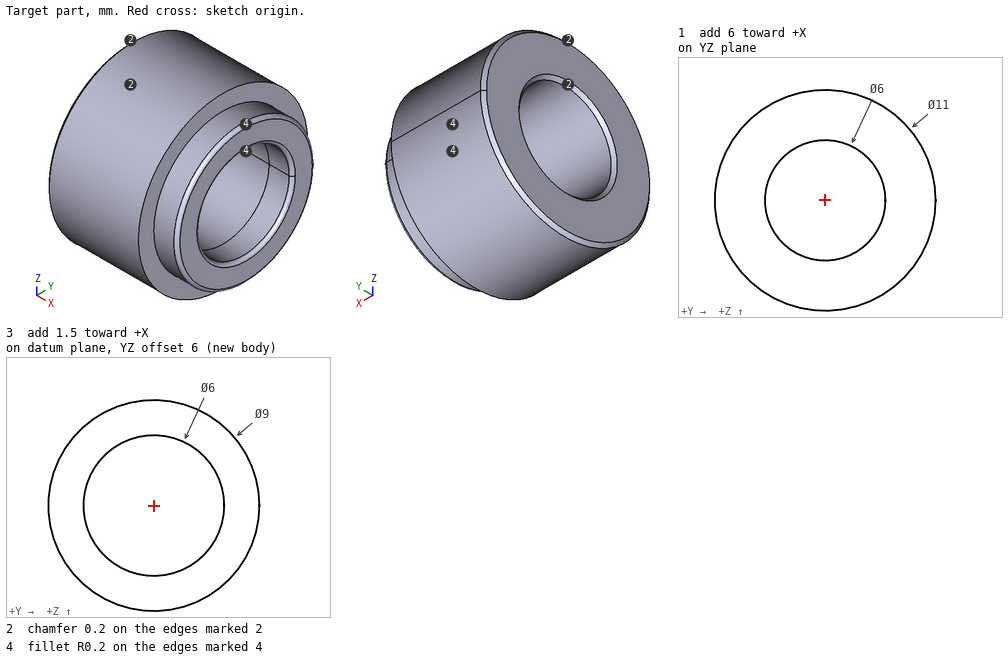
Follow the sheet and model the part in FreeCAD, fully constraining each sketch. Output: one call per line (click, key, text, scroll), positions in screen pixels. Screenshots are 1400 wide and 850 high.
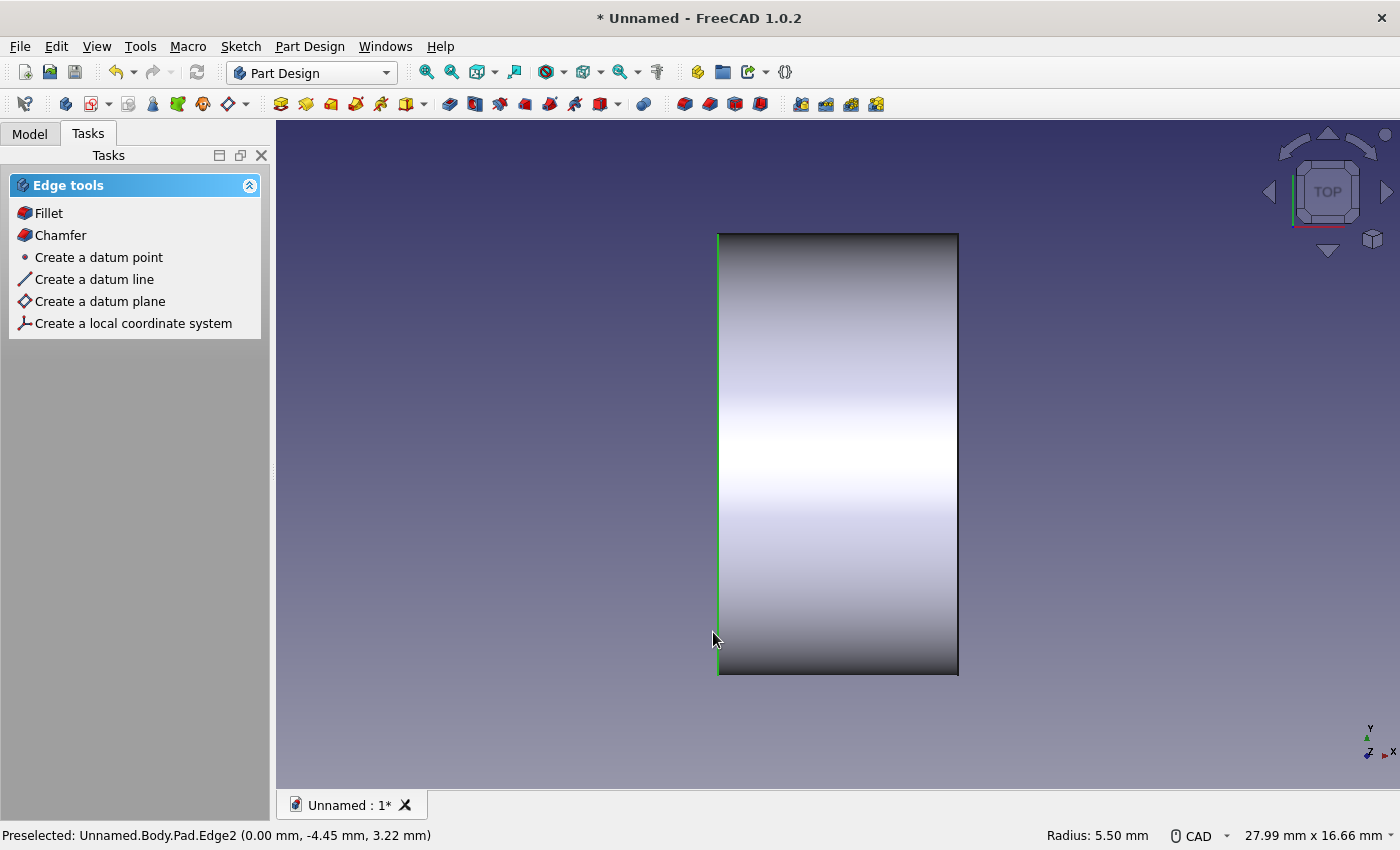
key(1)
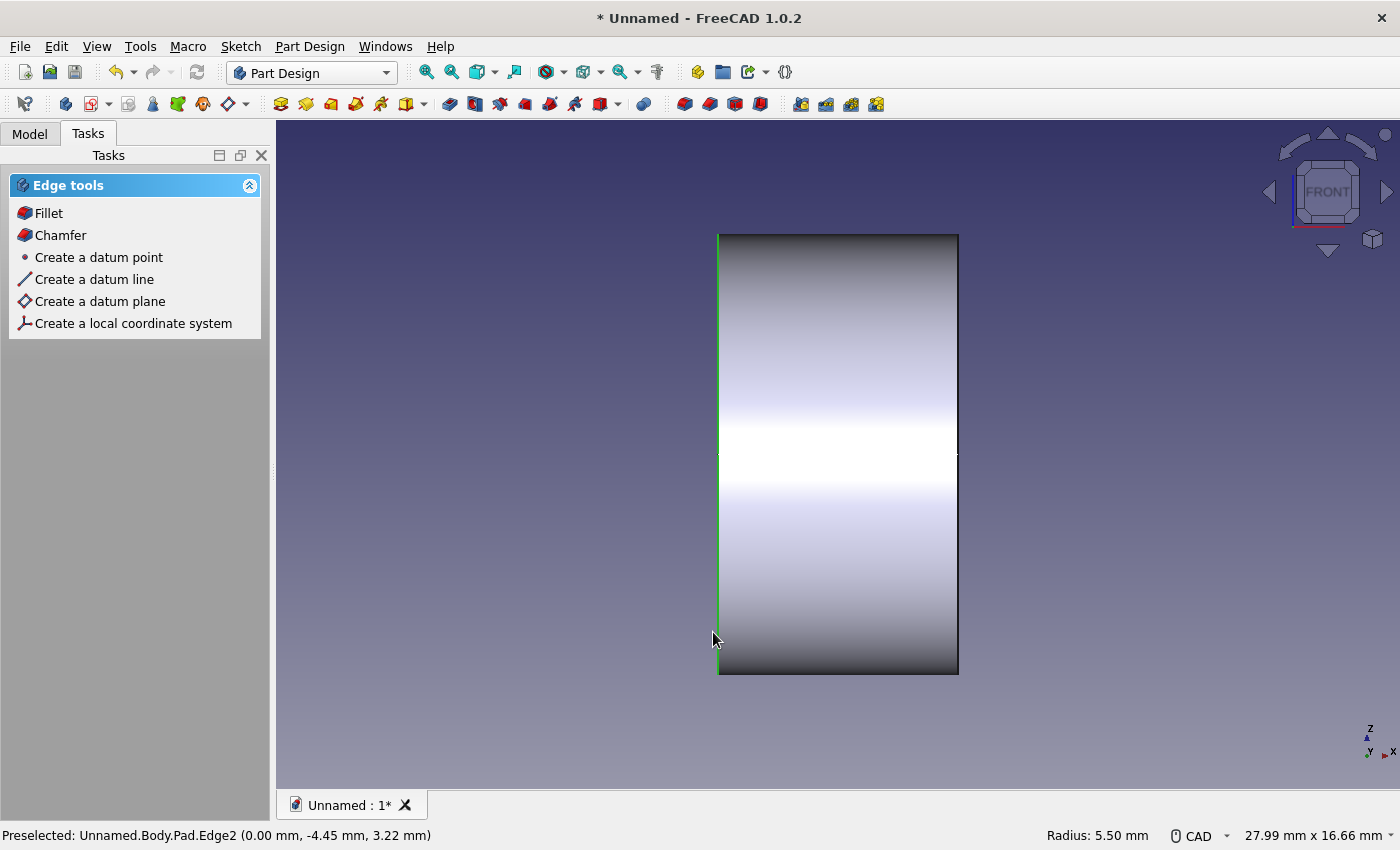
key(3)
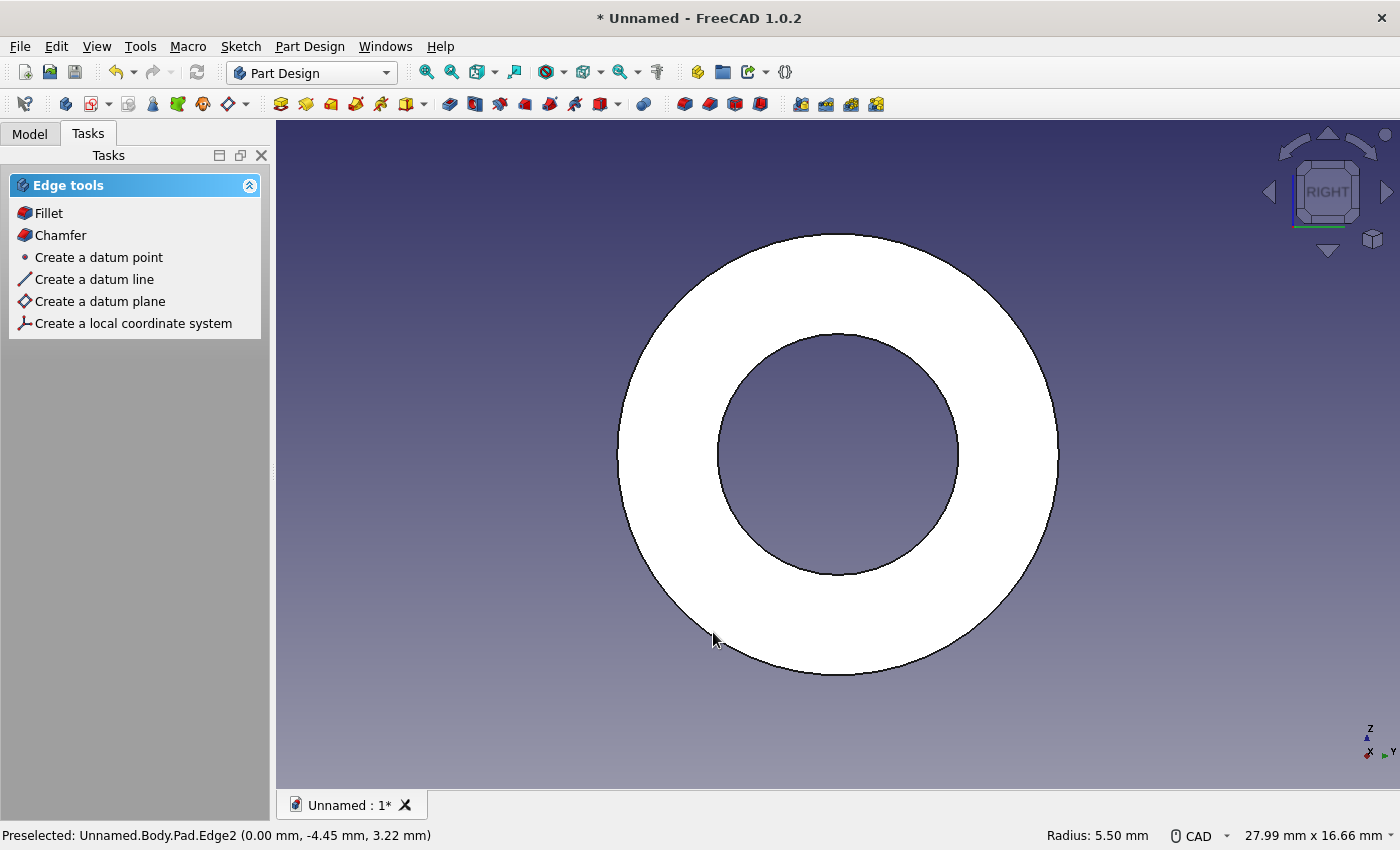
key(5)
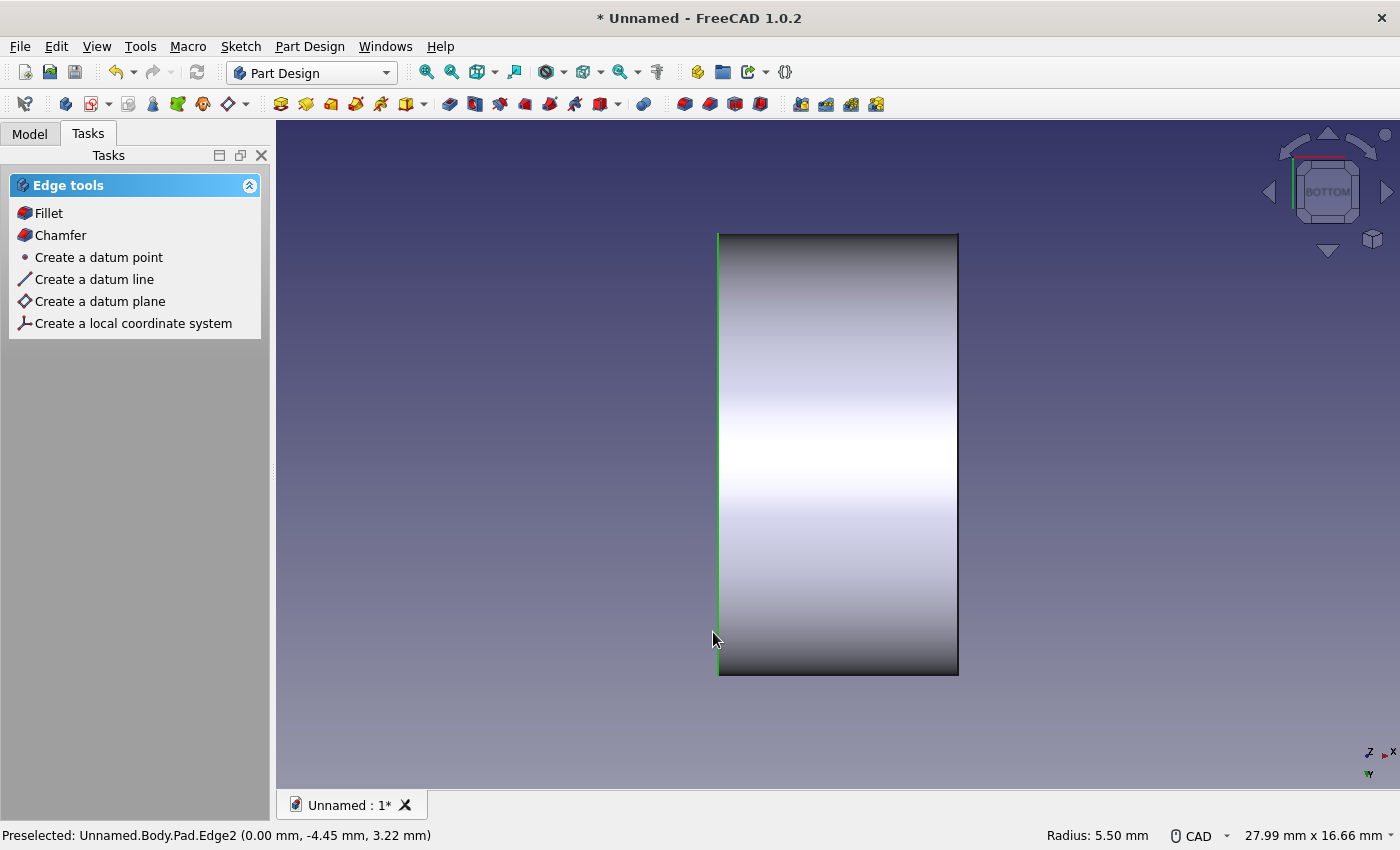
key(4)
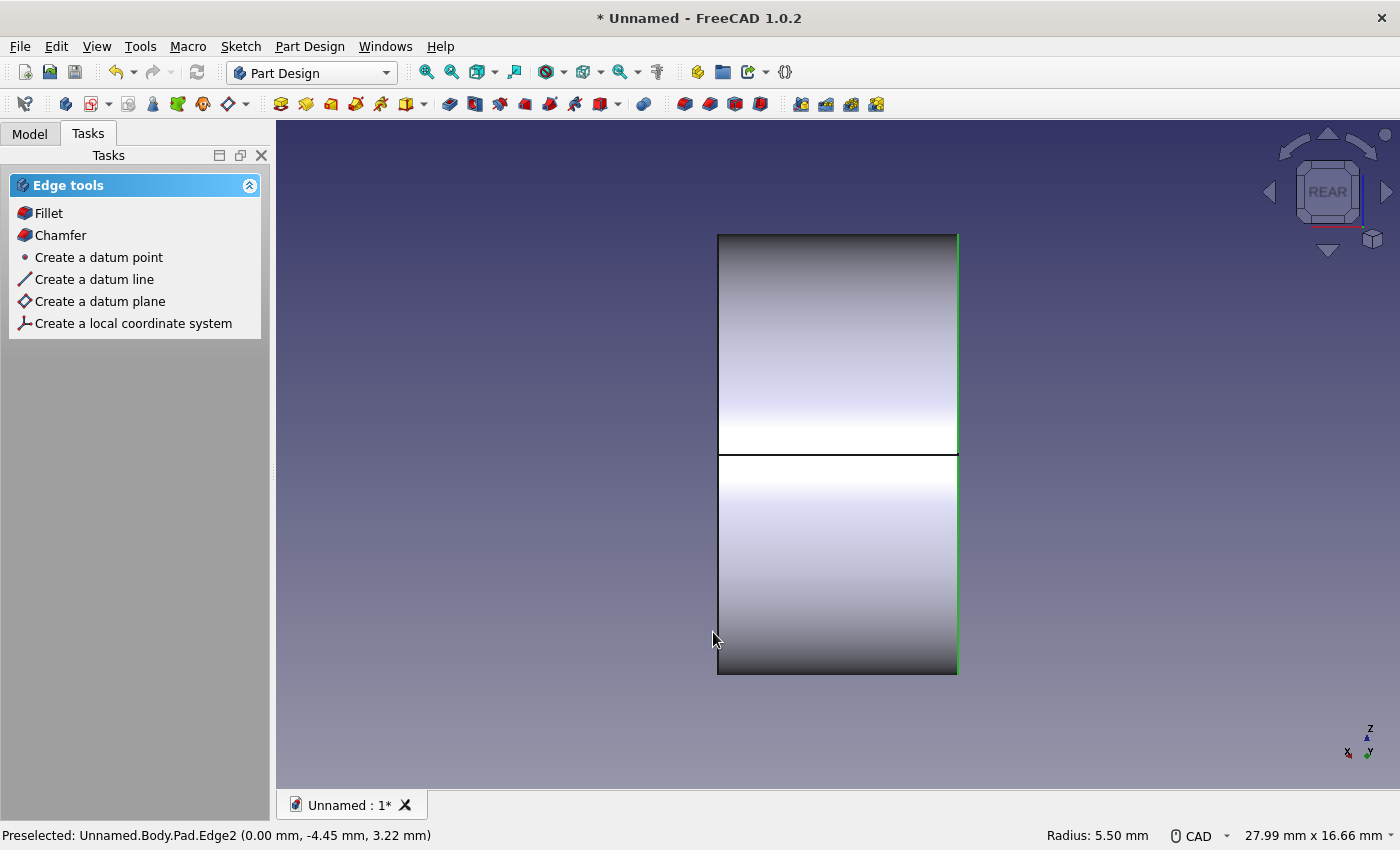
key(6)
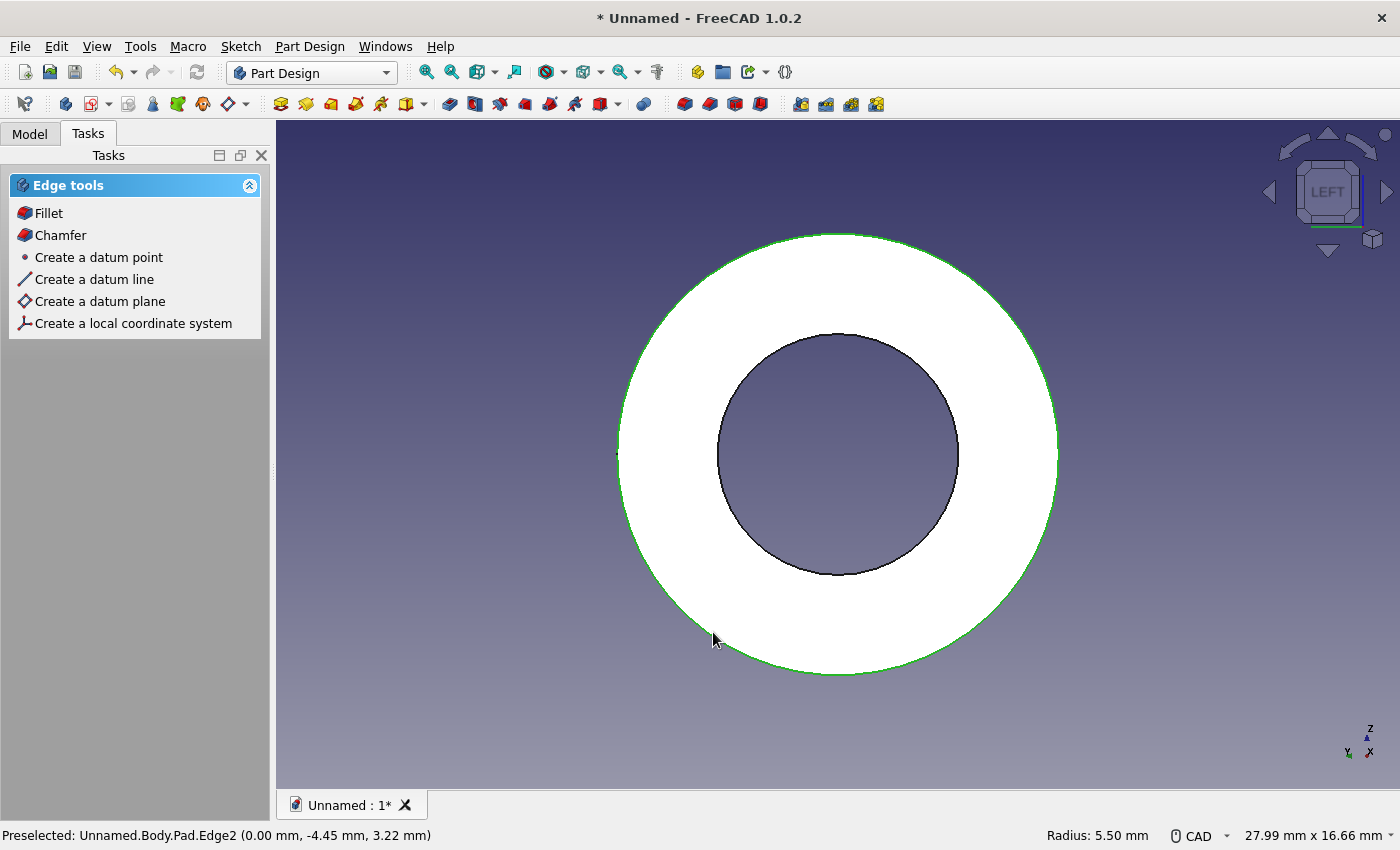
click(958, 453, ctrl)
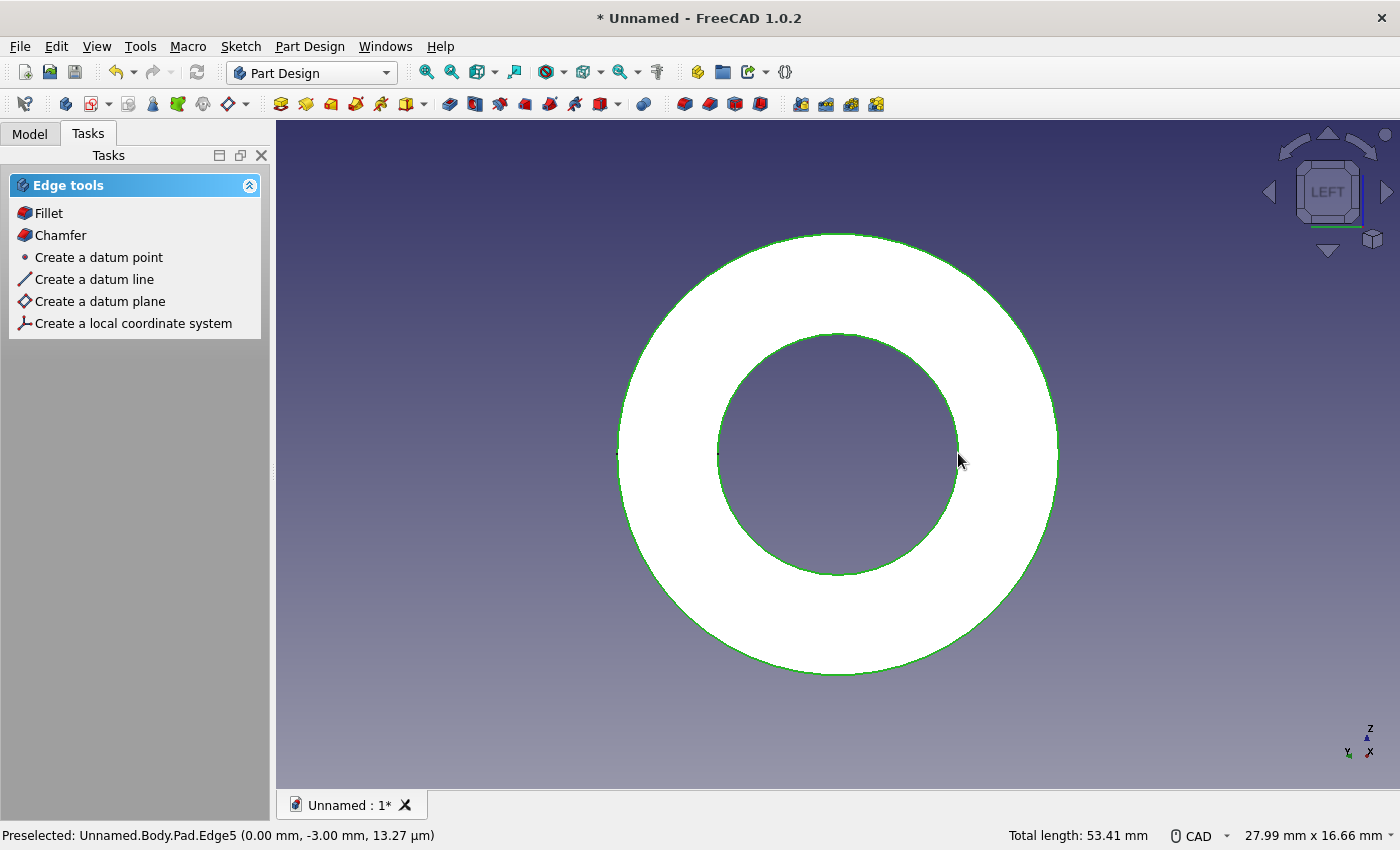
click(710, 104)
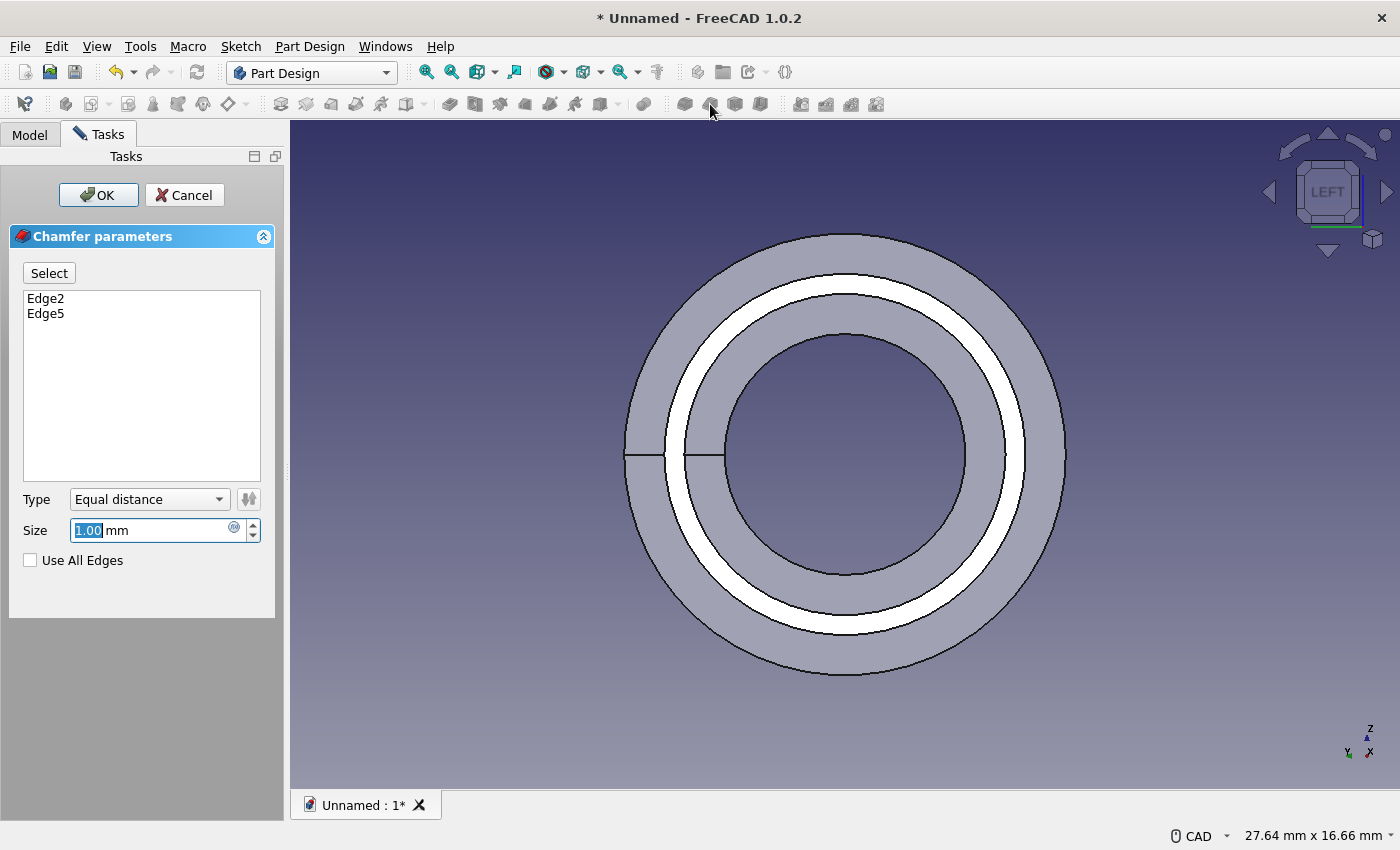
text(0.2)
key(Tab)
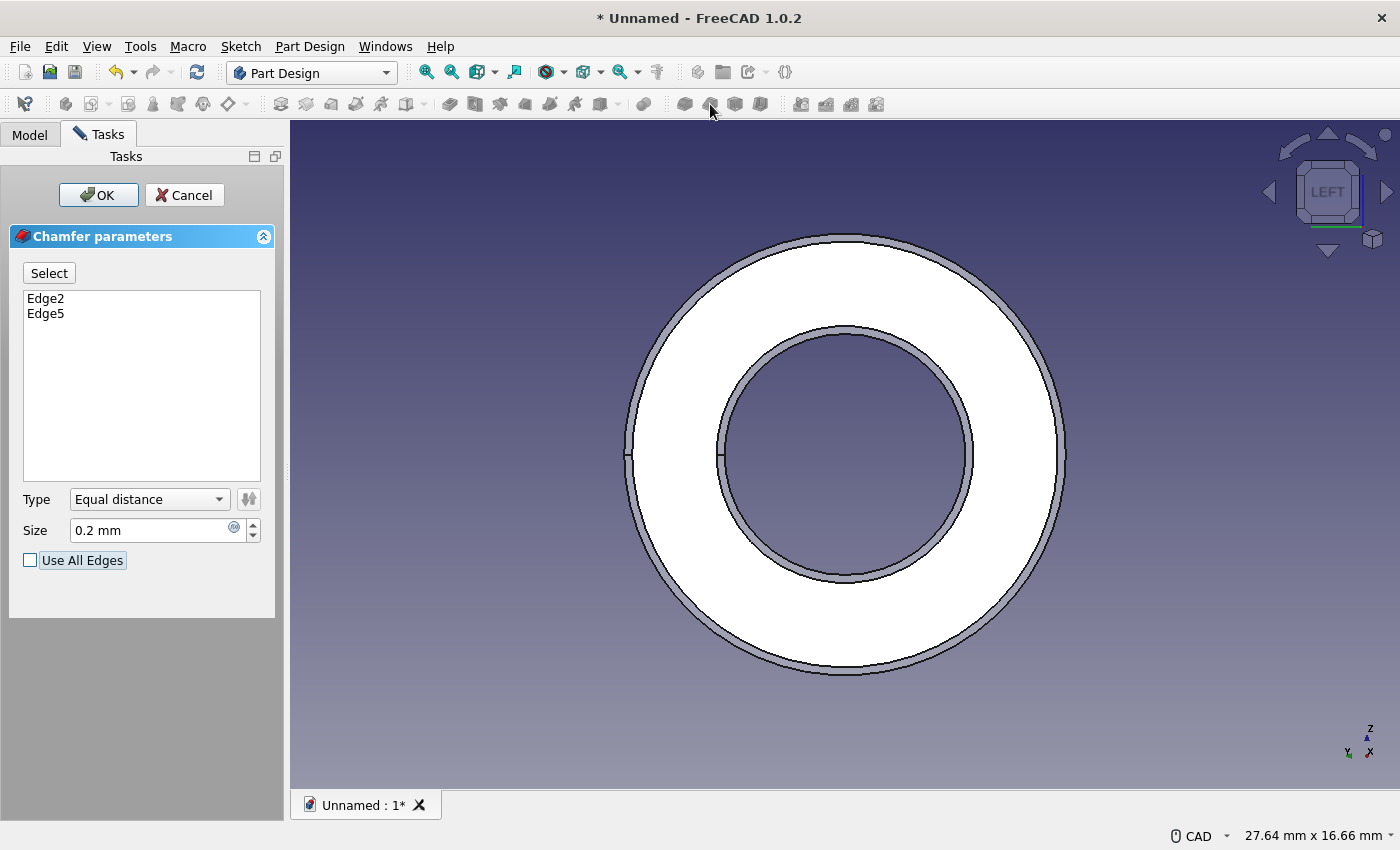
click(99, 195)